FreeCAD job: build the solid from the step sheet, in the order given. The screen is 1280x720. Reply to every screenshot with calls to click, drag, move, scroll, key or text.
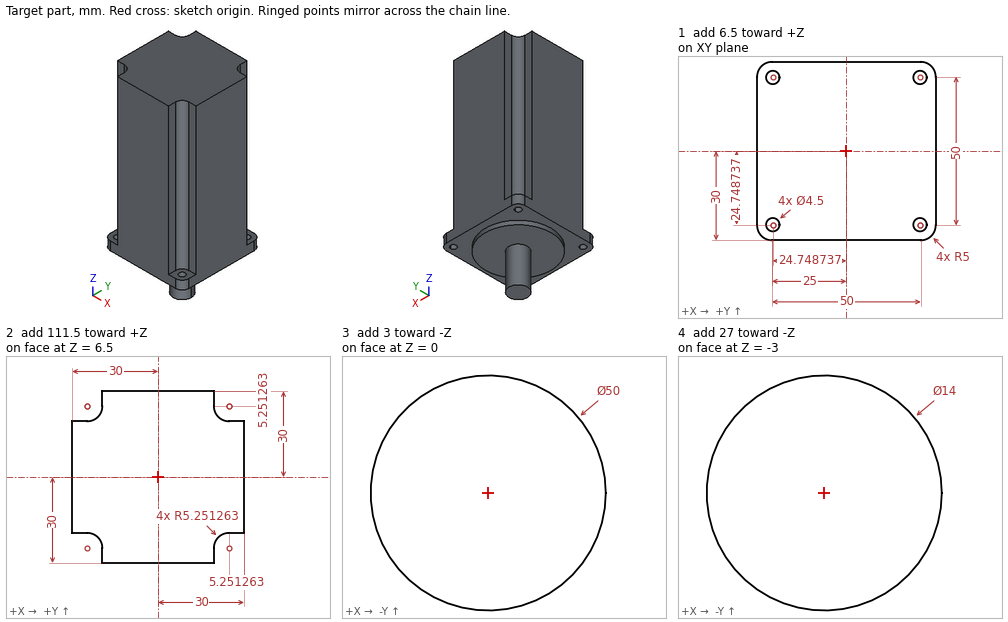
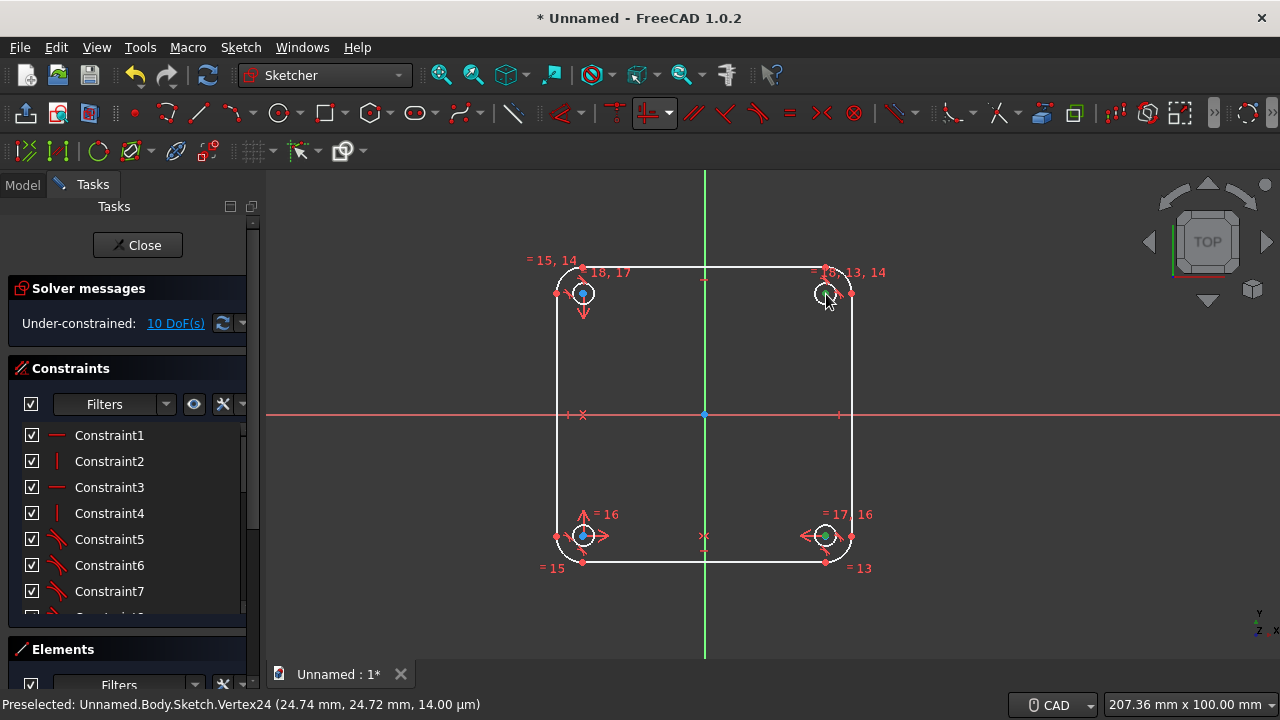
click(353, 415)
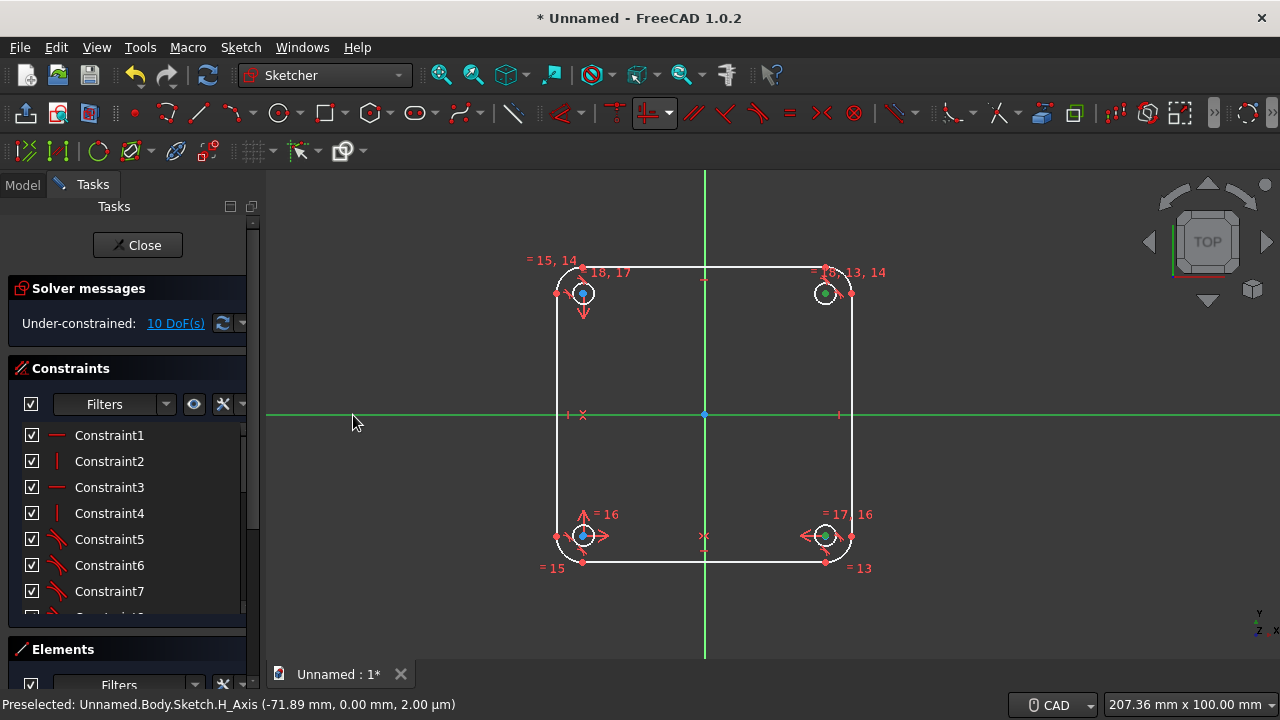
key(s)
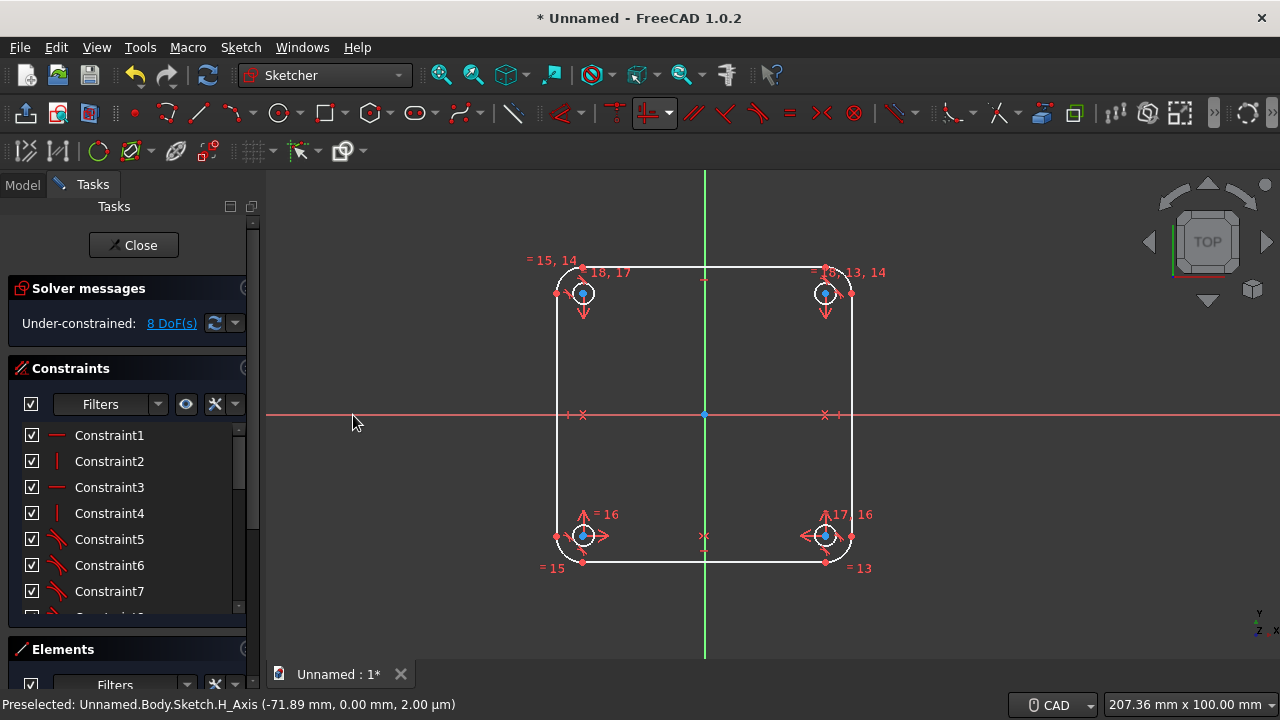
scroll(837, 560, up, 3)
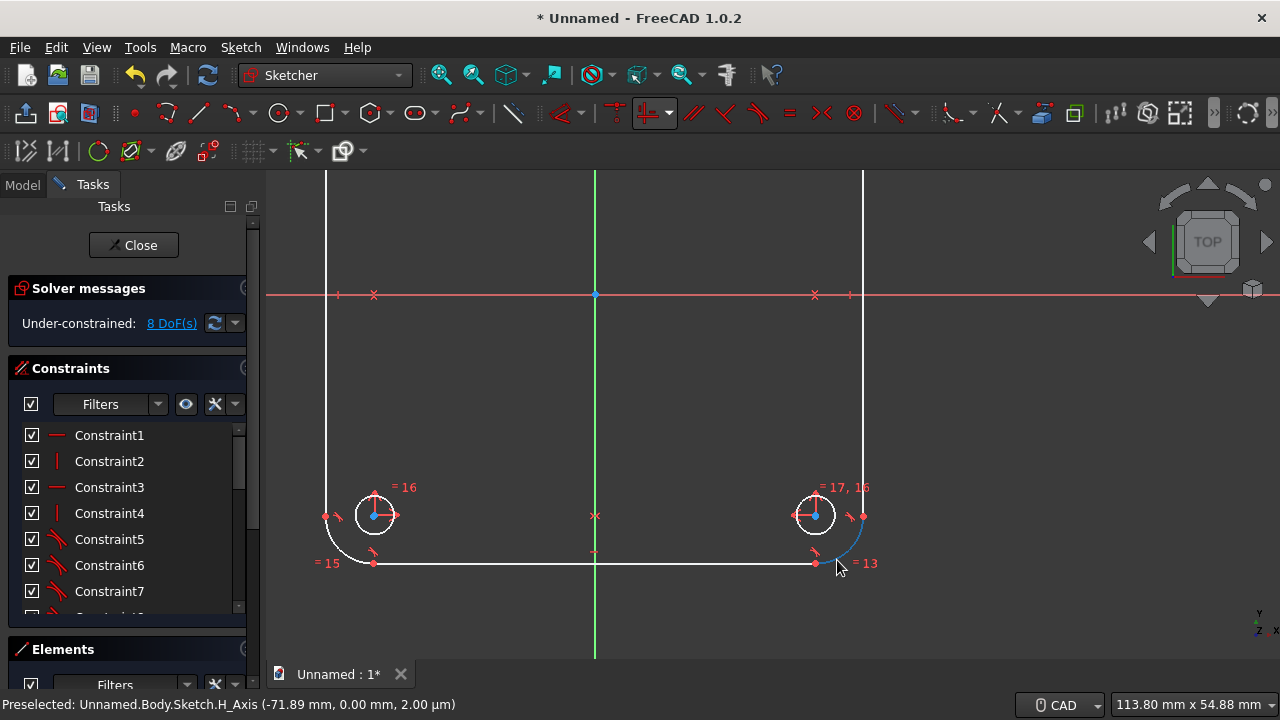
click(837, 558)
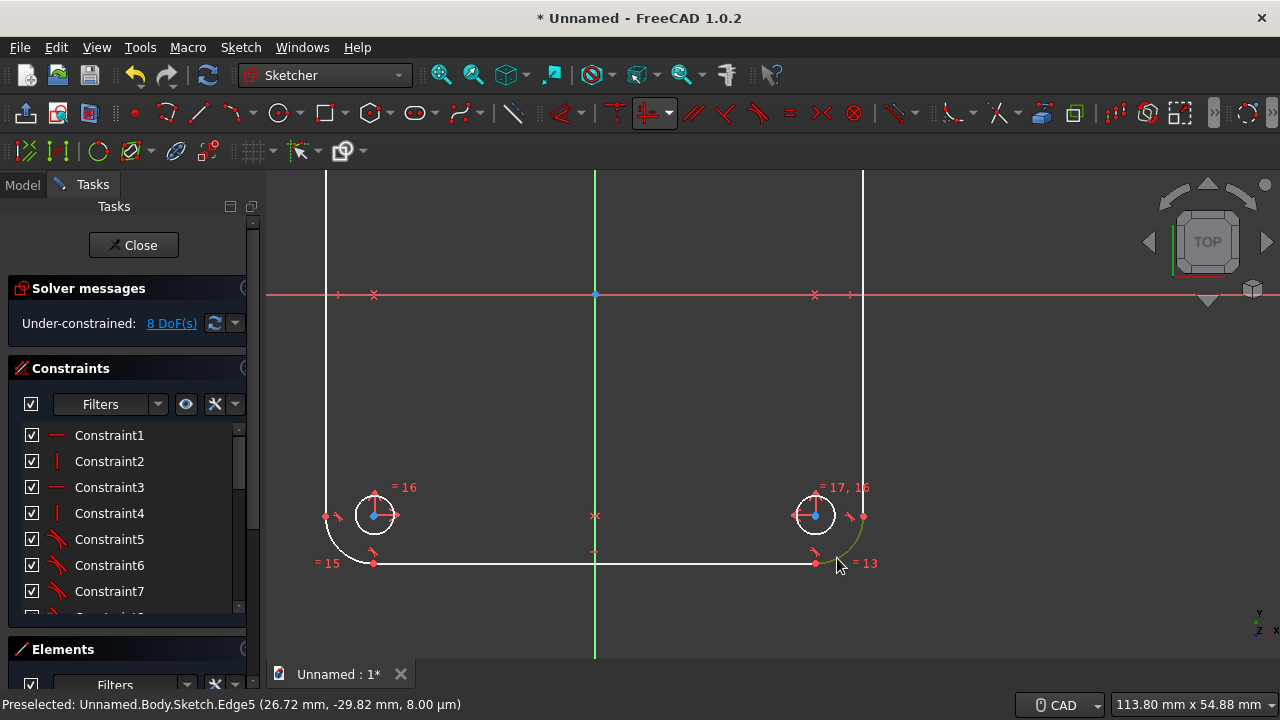
click(584, 114)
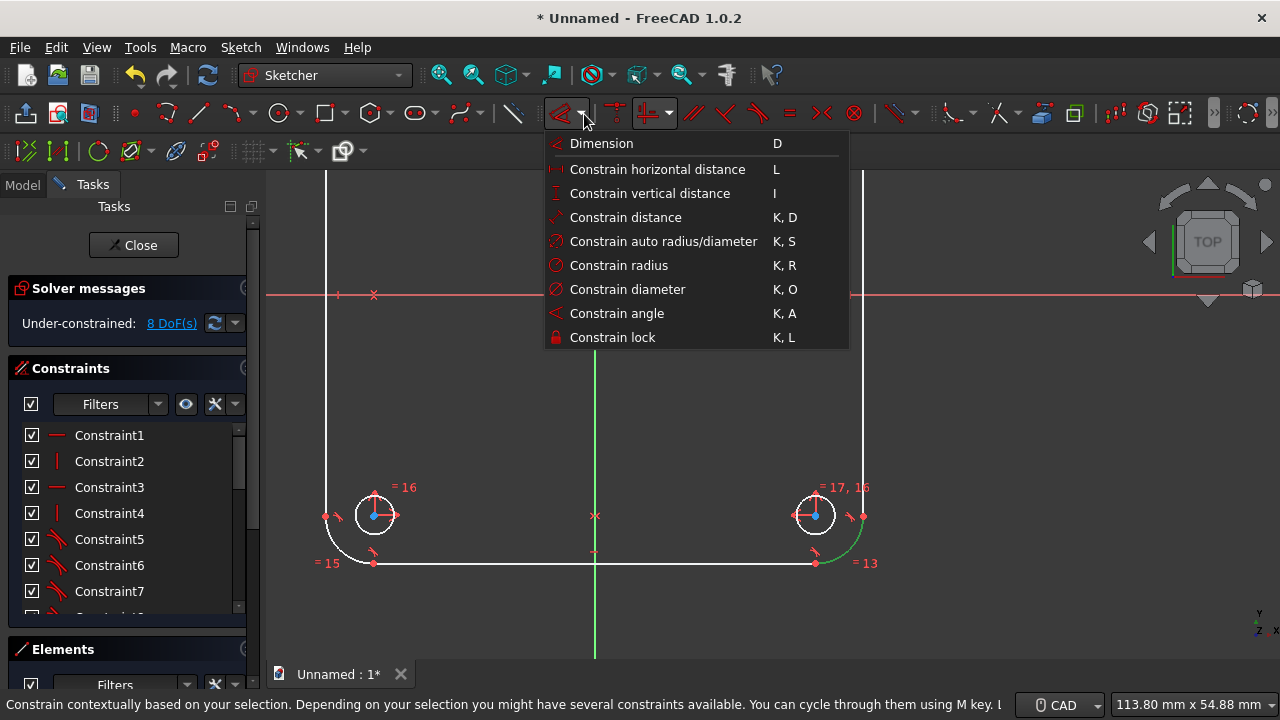
click(697, 265)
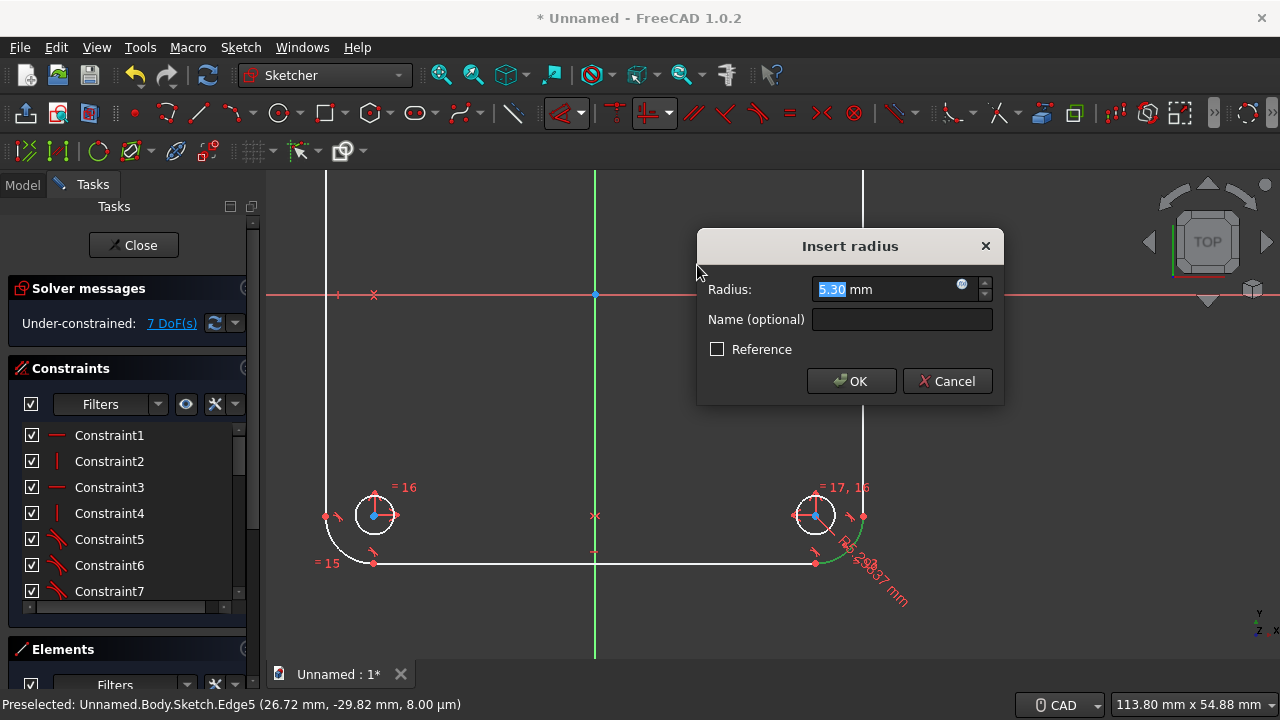
text(5)
key(Return)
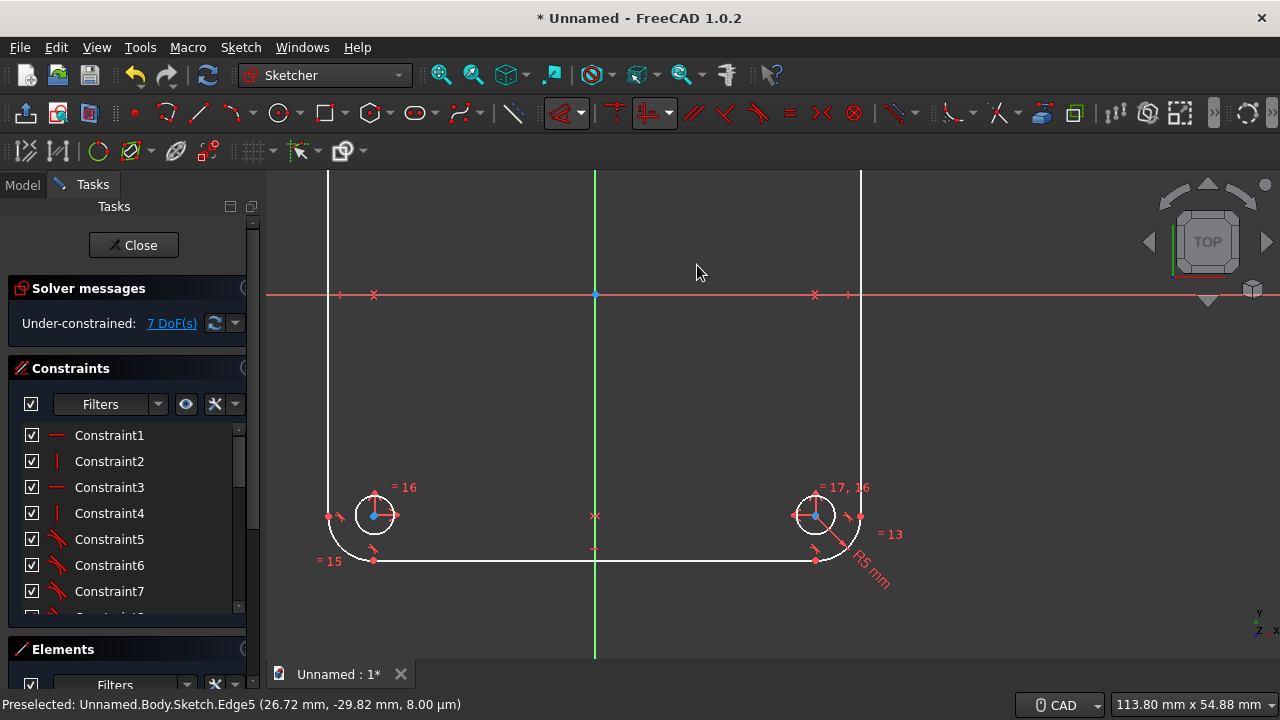
click(388, 502)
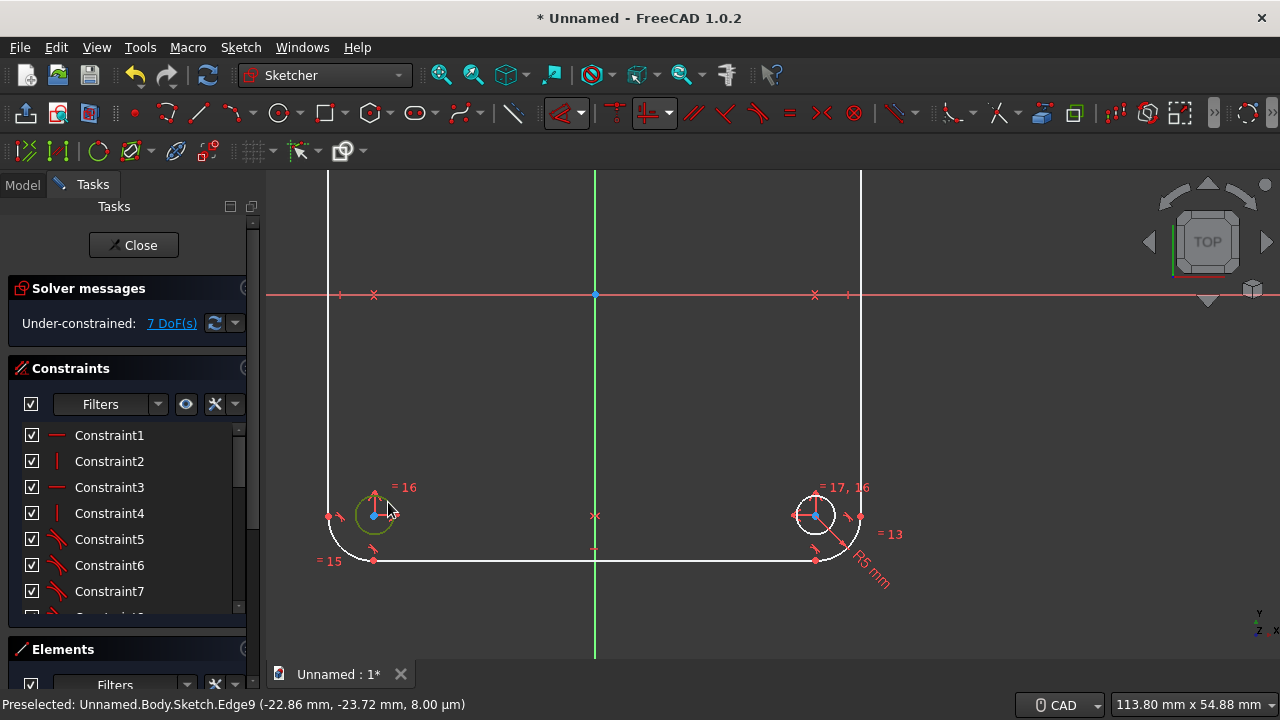
key(k)
key(o)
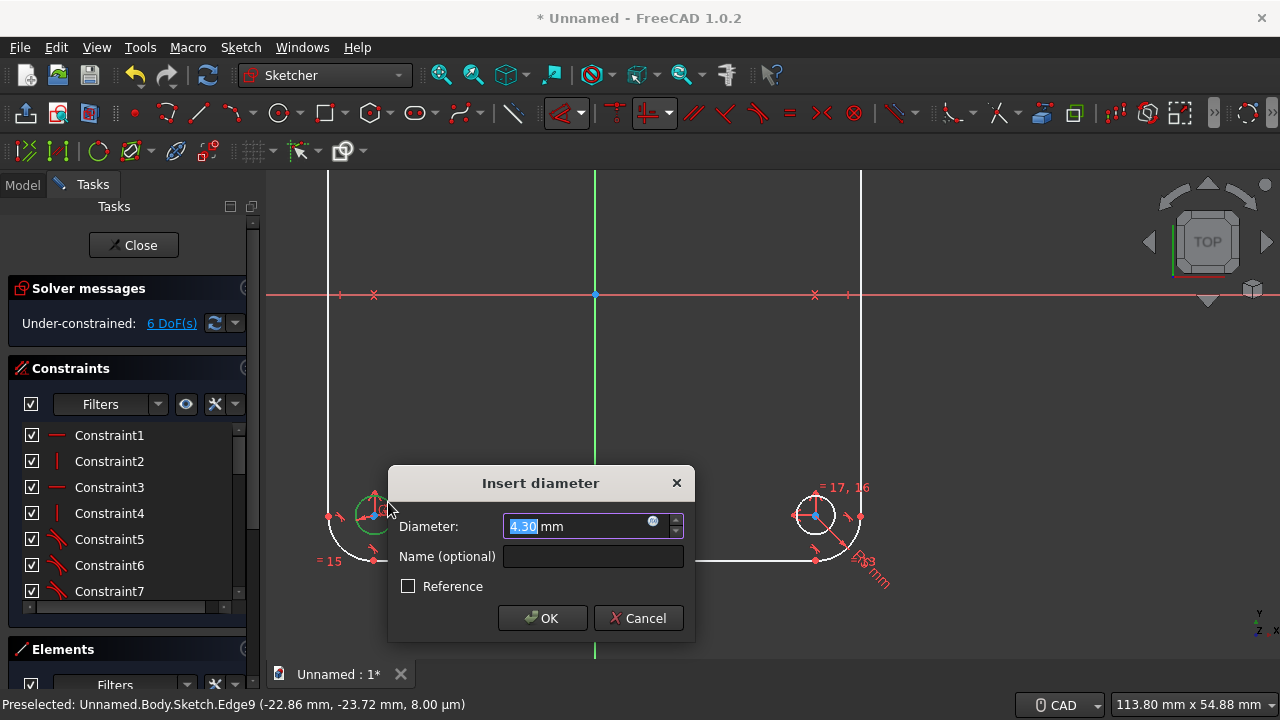
text(4.5)
key(Return)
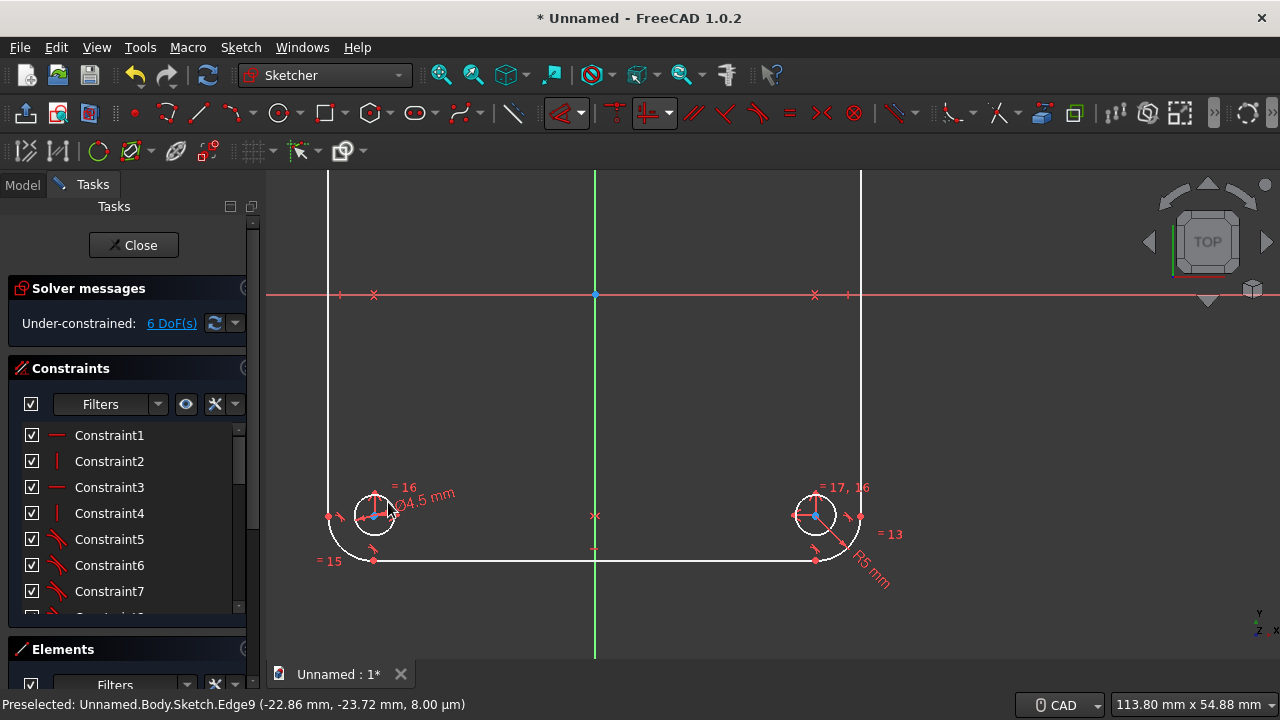
click(506, 561)